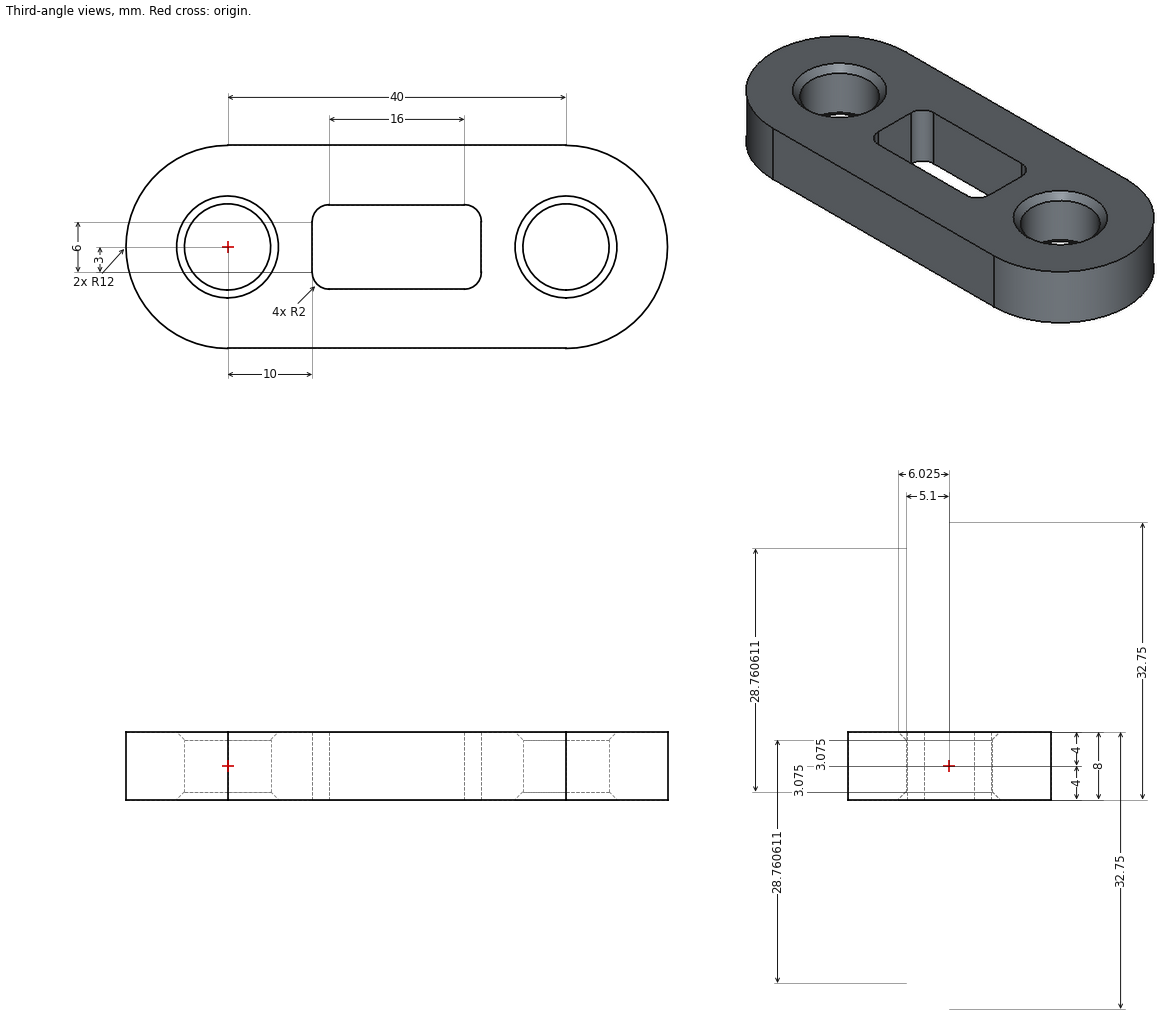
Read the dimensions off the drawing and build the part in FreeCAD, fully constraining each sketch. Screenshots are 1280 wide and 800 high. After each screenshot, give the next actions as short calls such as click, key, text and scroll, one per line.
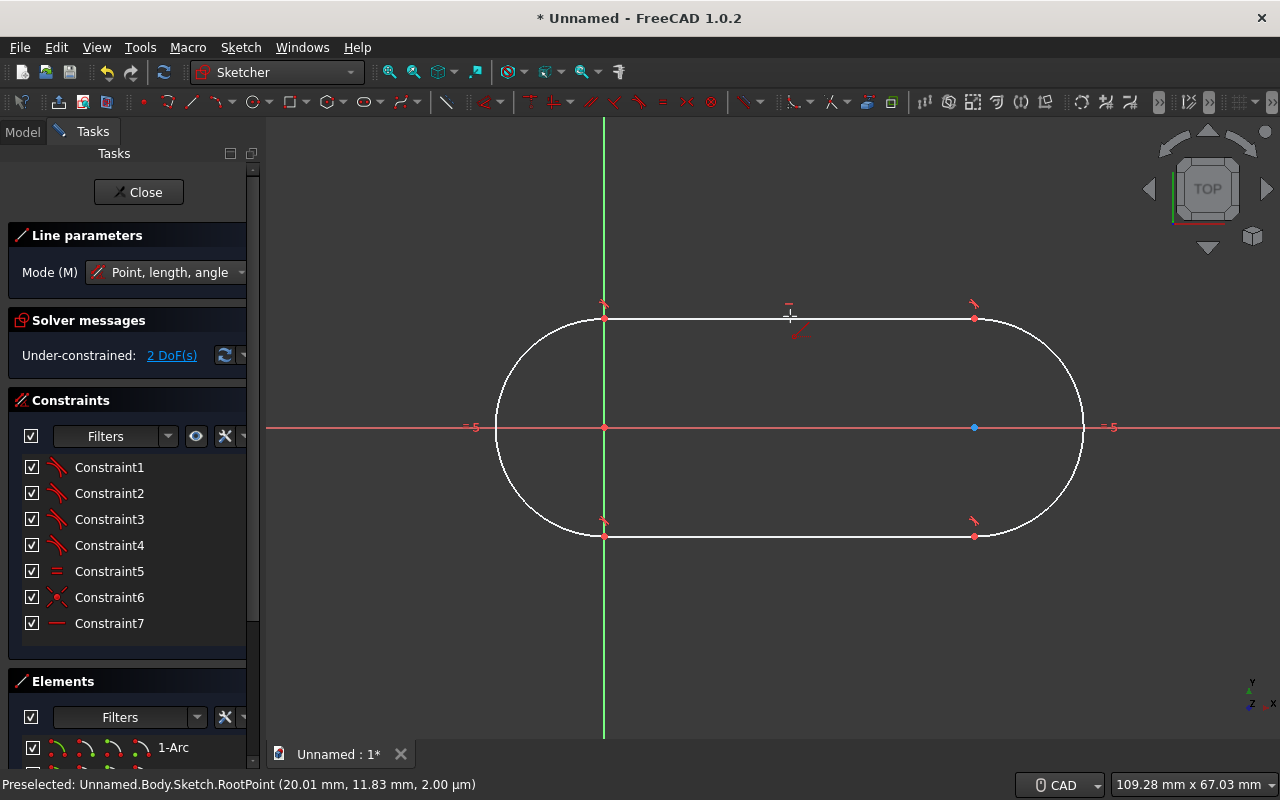
click(697, 456)
click(697, 400)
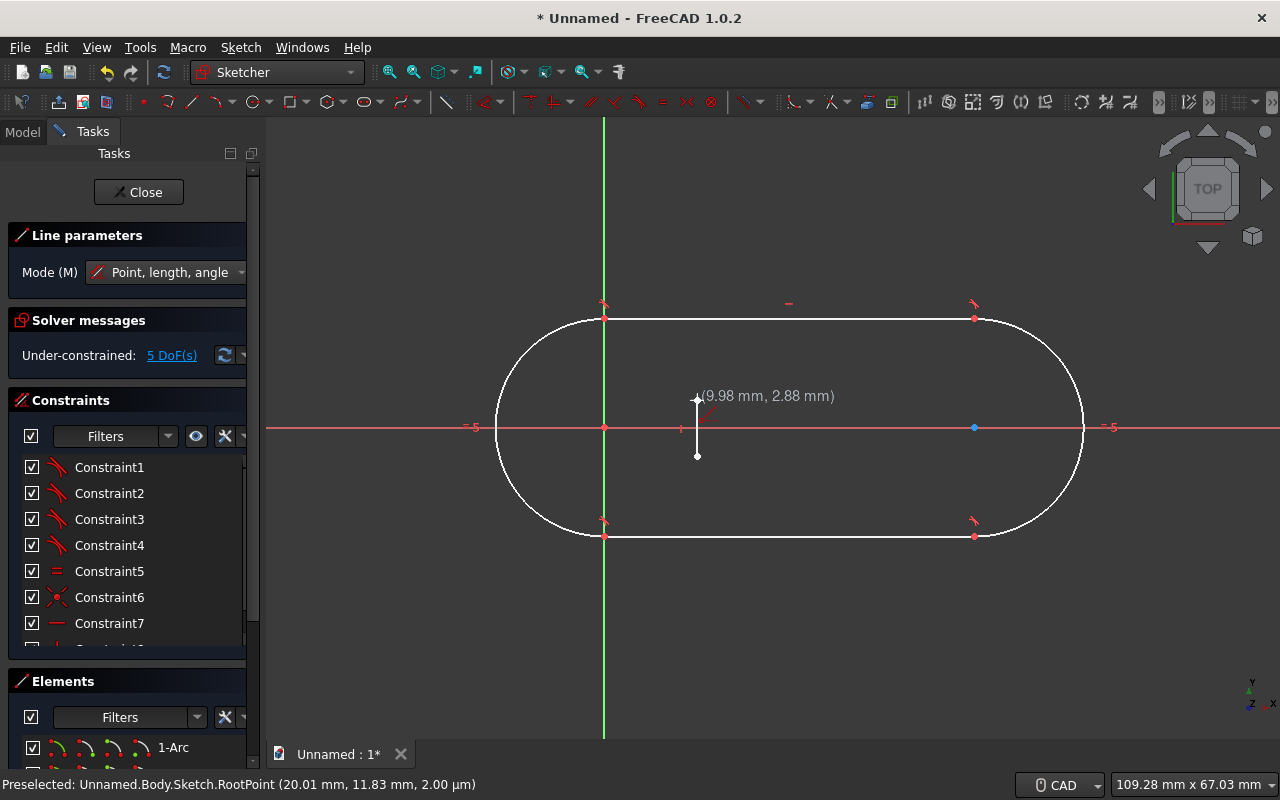
click(716, 381)
click(864, 381)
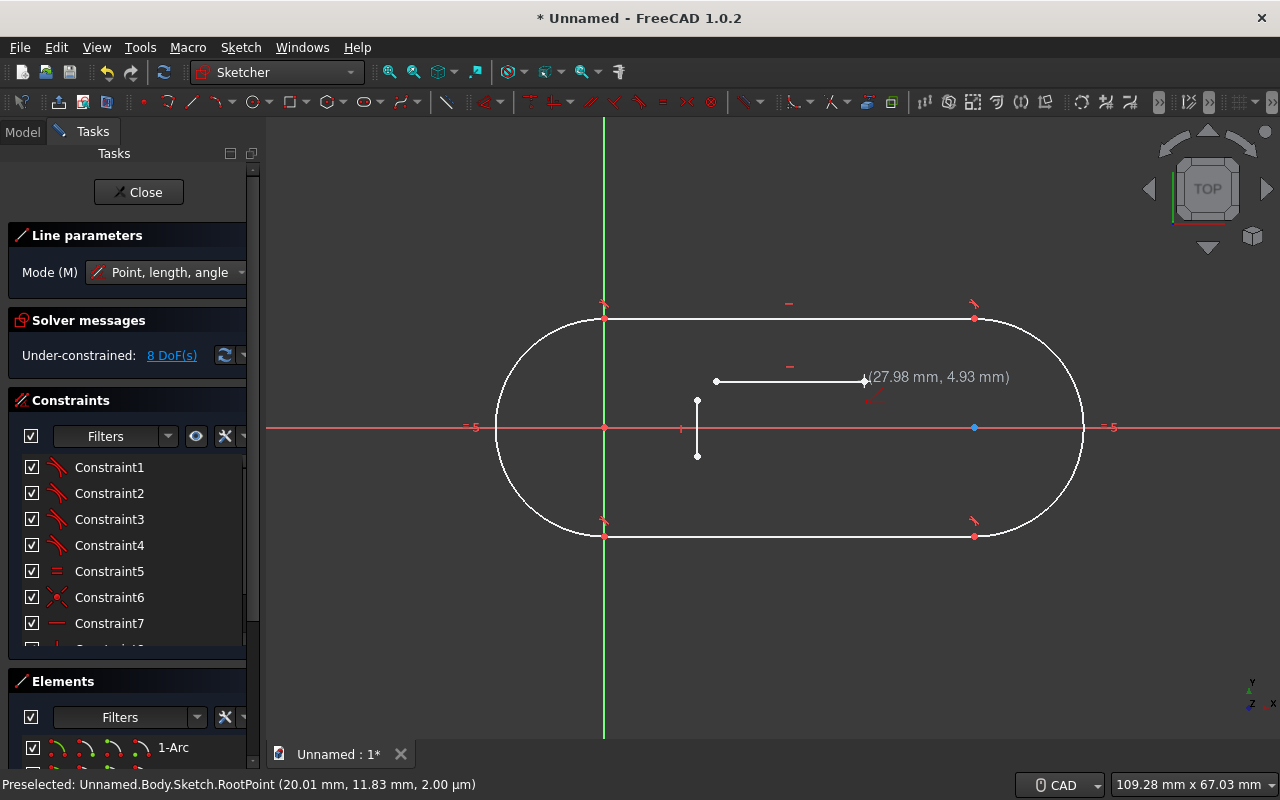
click(883, 400)
click(883, 456)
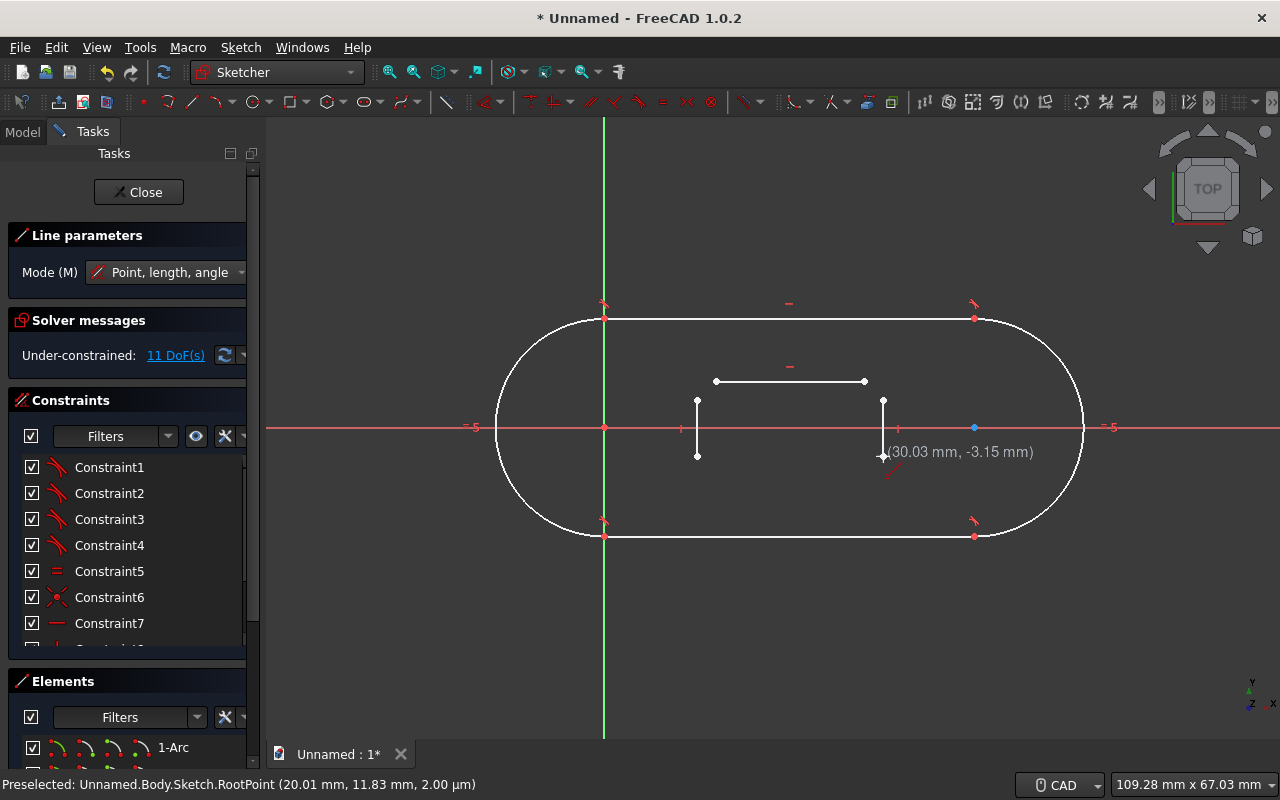
click(864, 474)
click(716, 474)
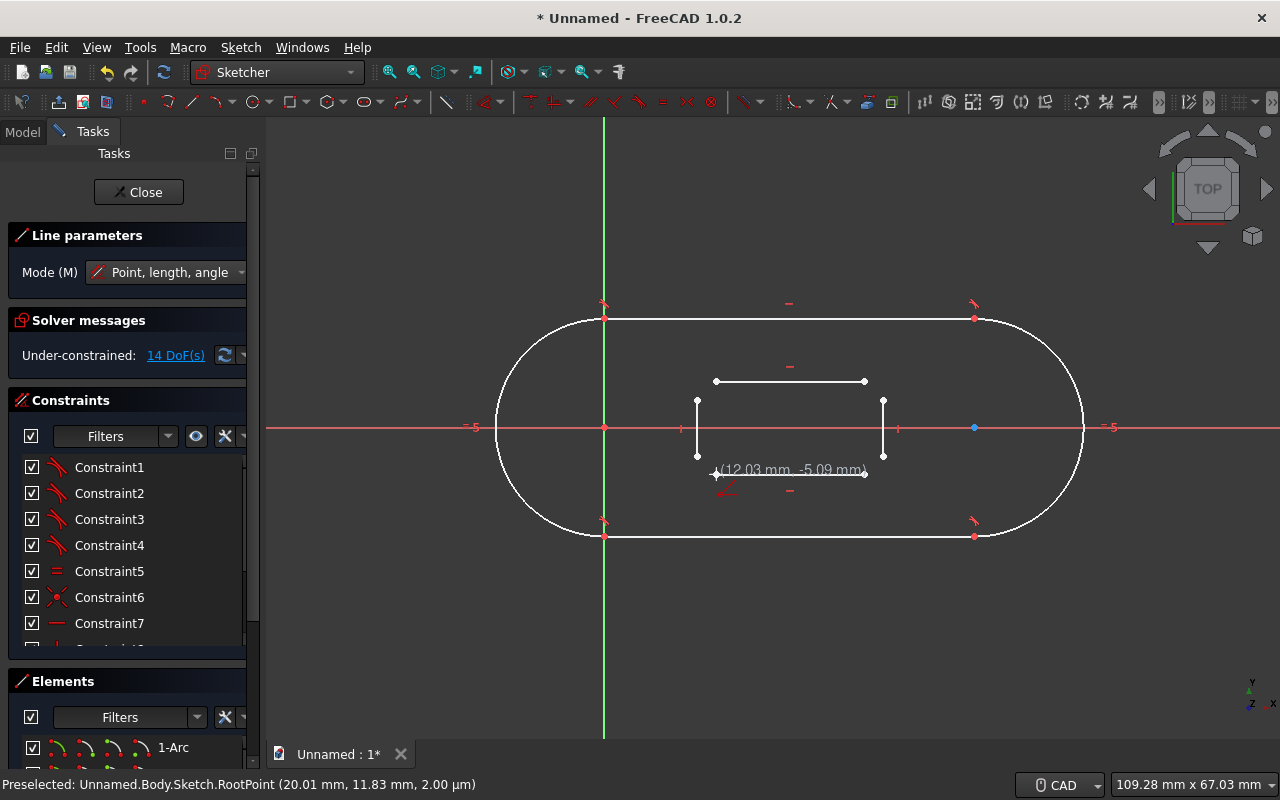
key(g)
key(3)
key(a)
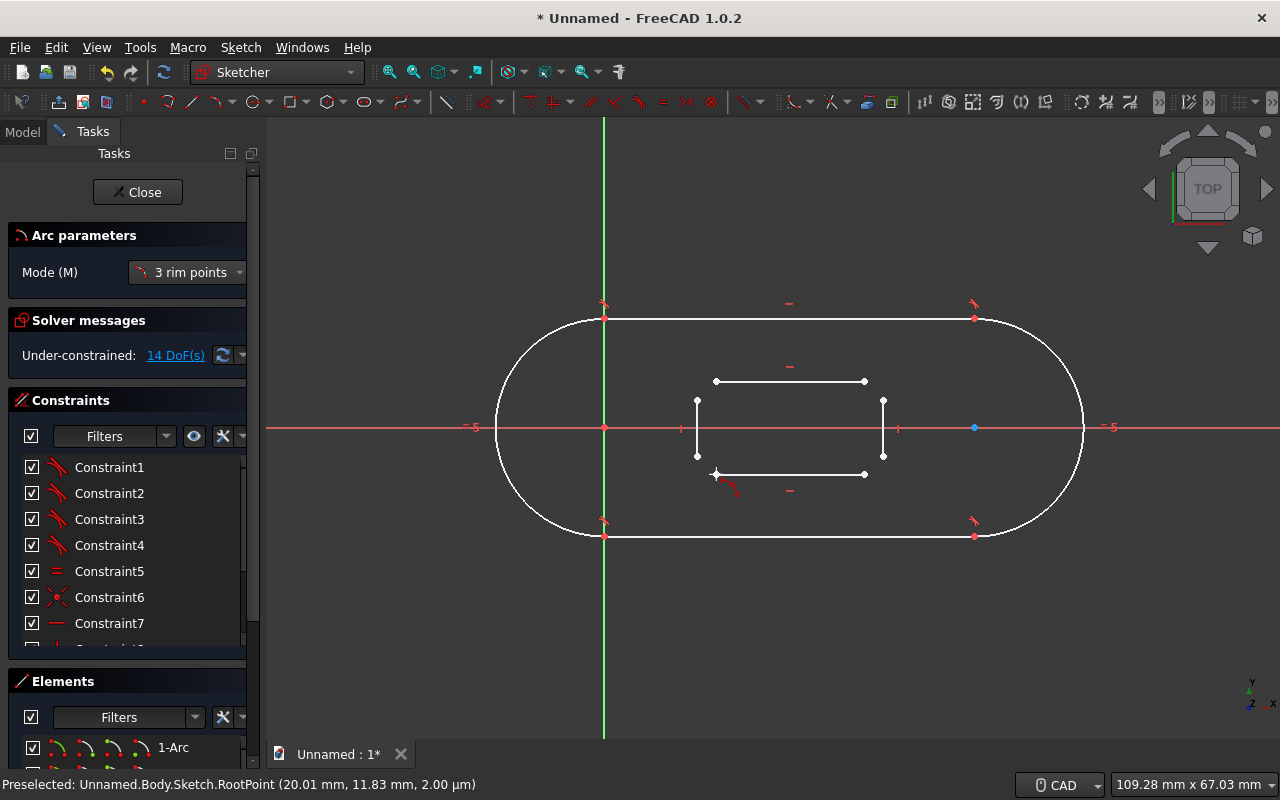
click(697, 401)
click(716, 382)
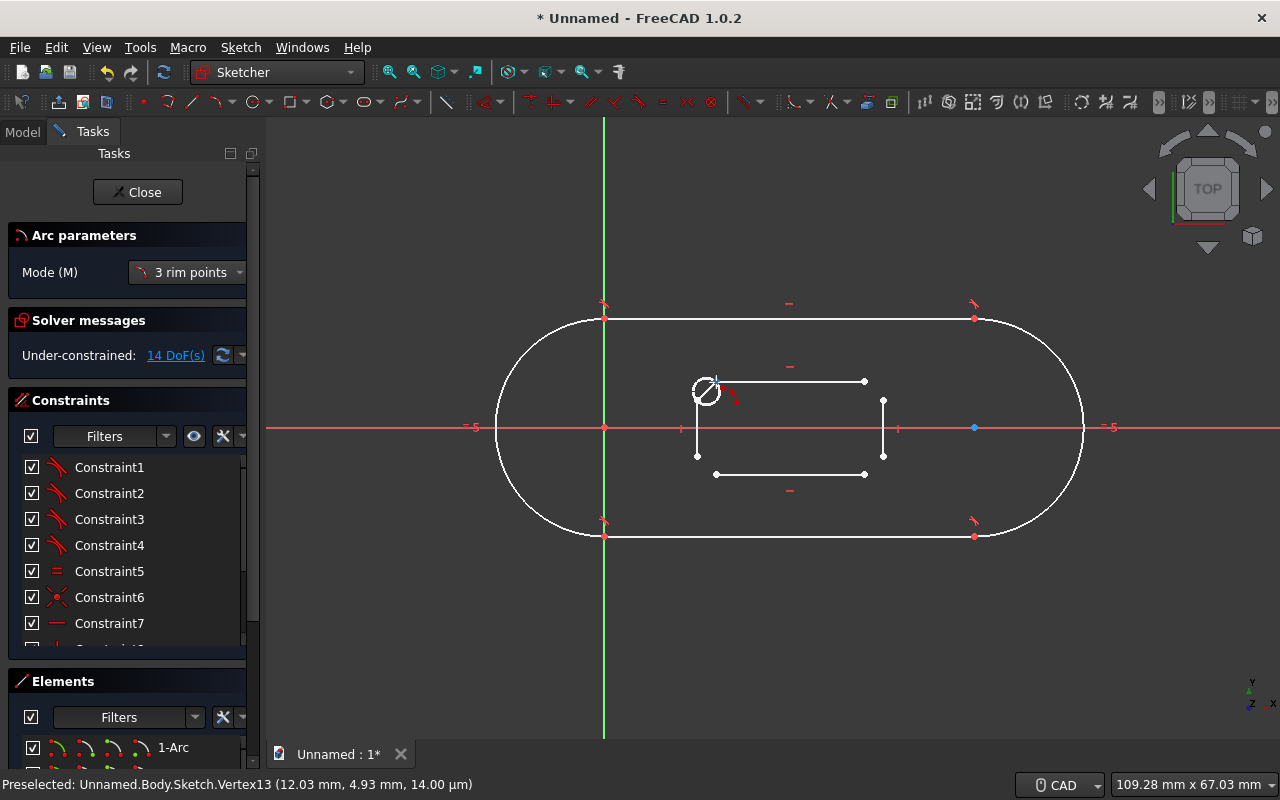
scroll(703, 387, up, 6)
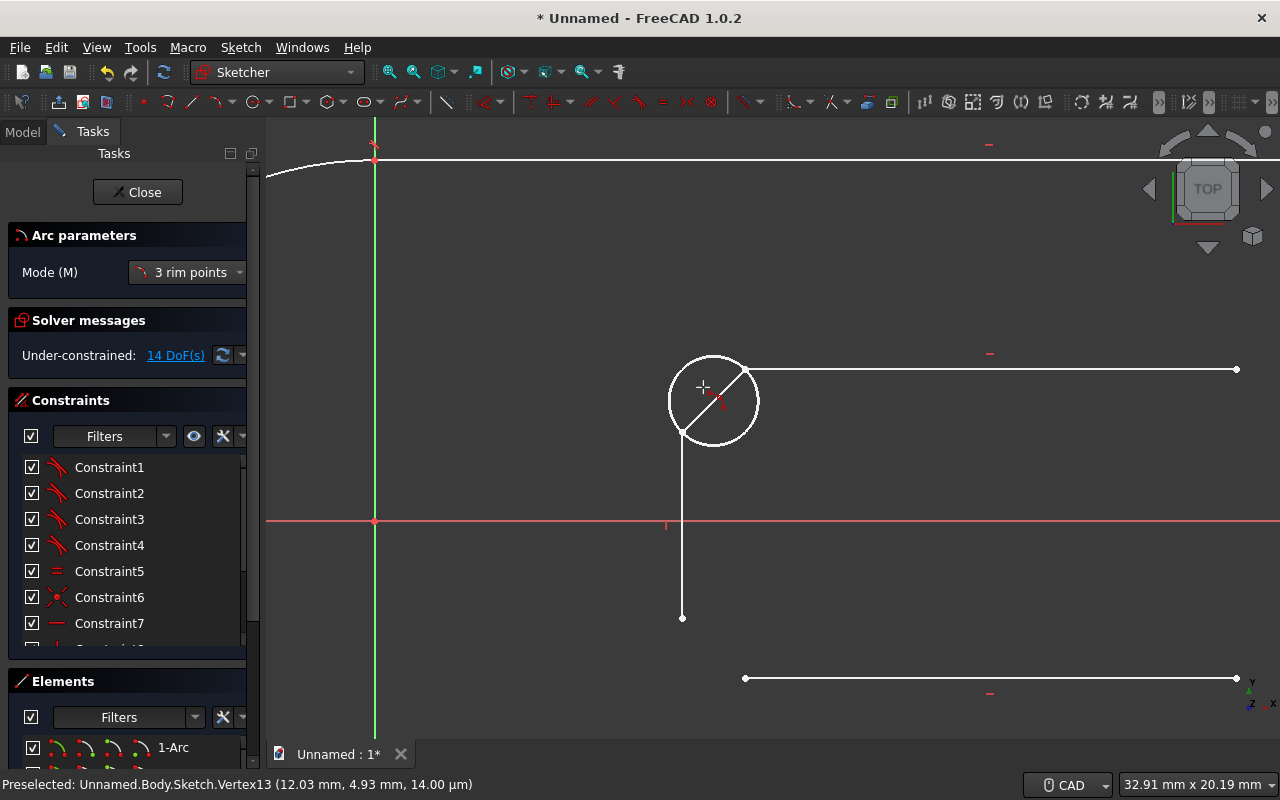
click(701, 385)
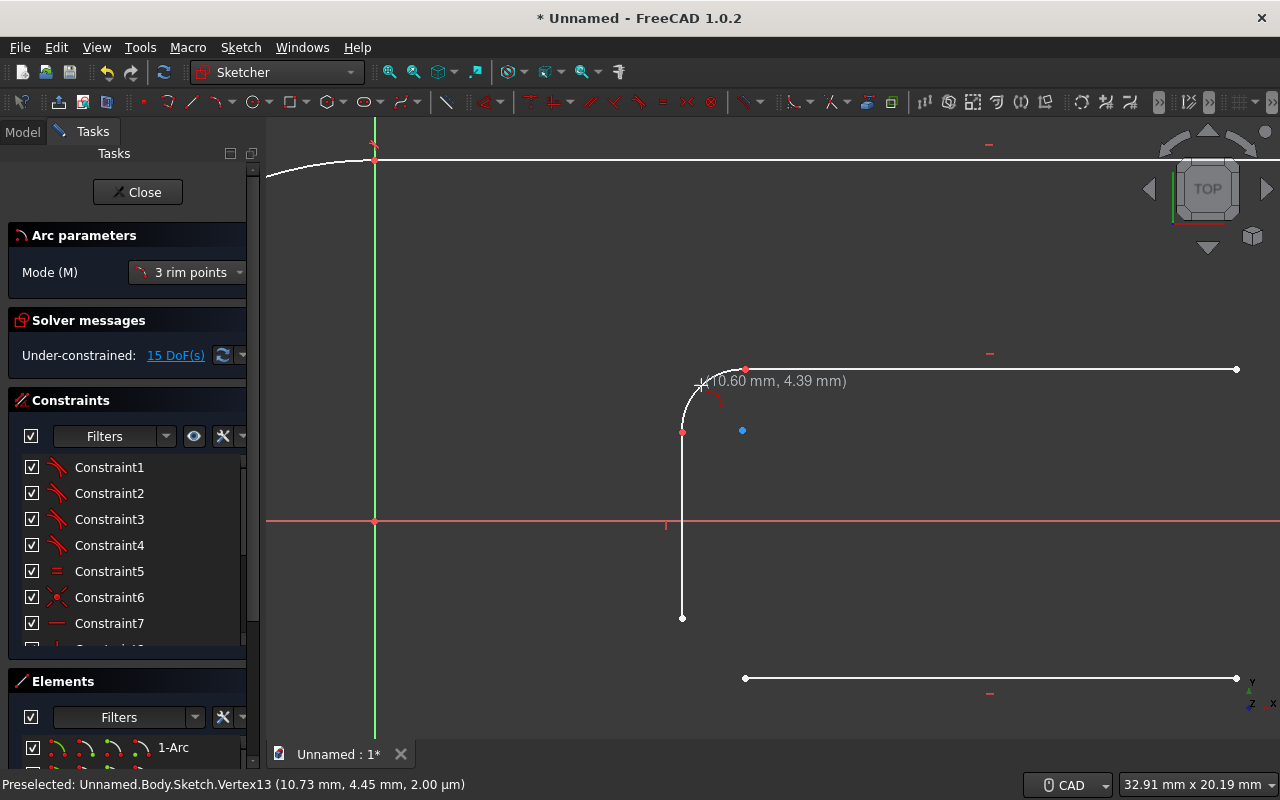
scroll(581, 388, down, 6)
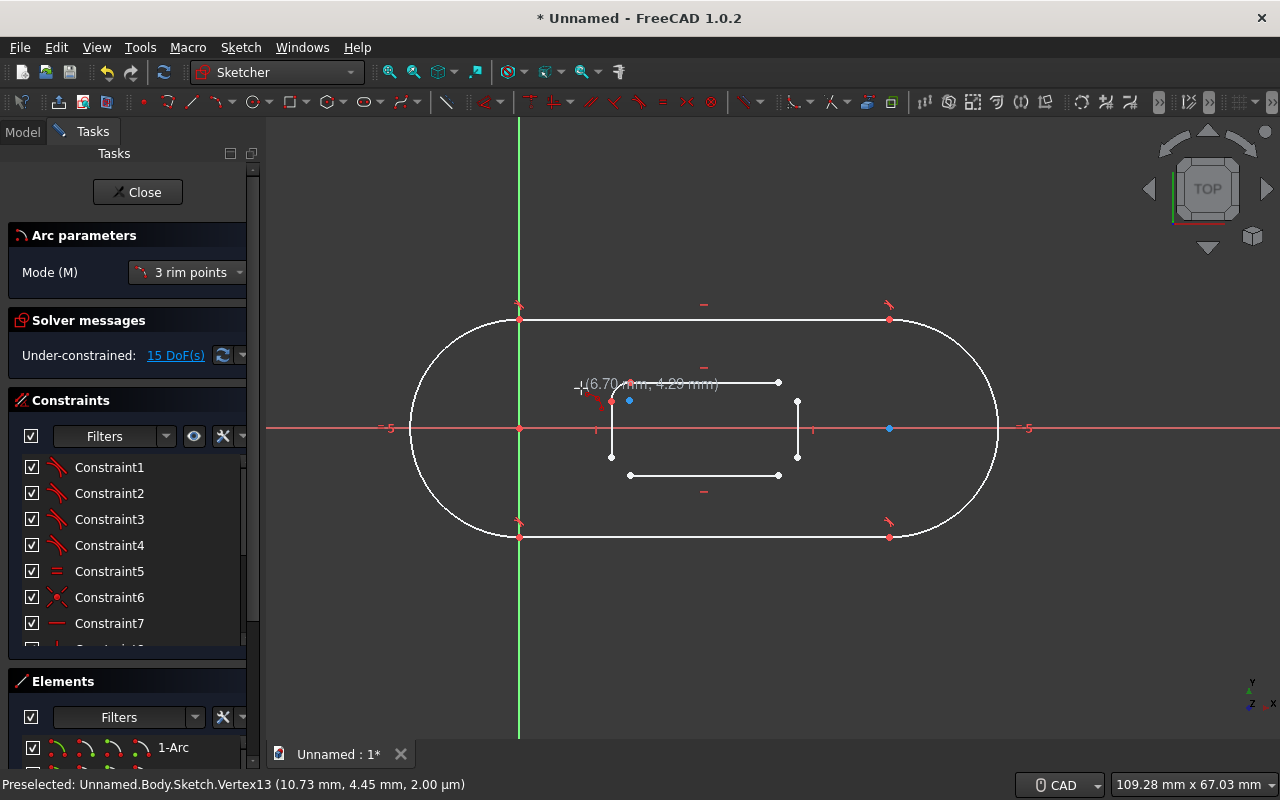
click(779, 383)
click(798, 402)